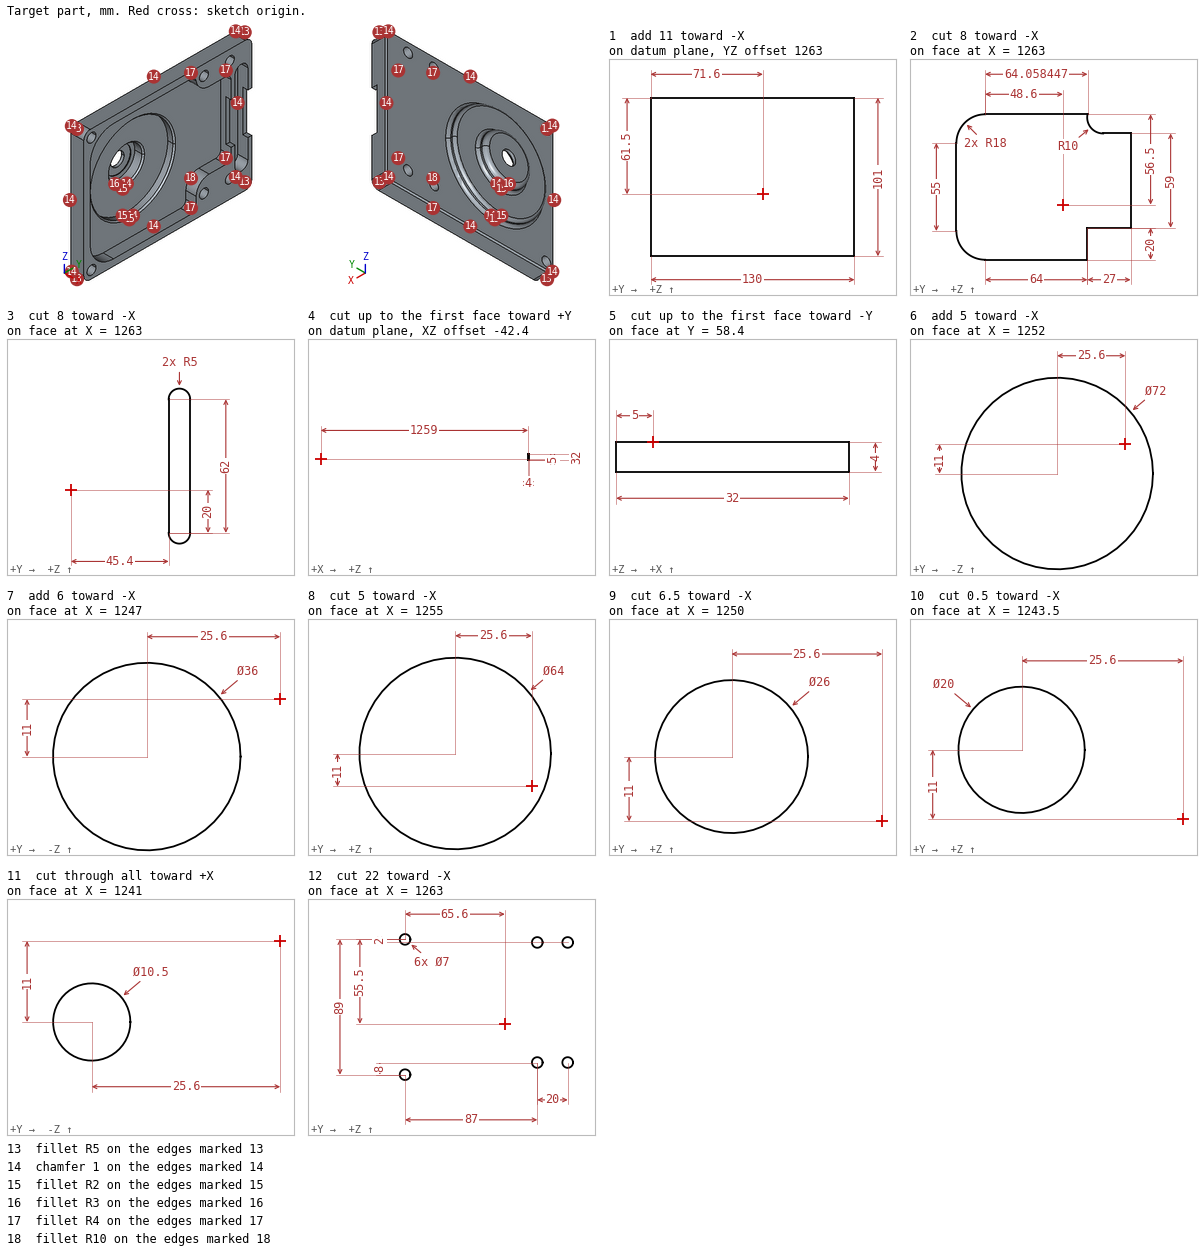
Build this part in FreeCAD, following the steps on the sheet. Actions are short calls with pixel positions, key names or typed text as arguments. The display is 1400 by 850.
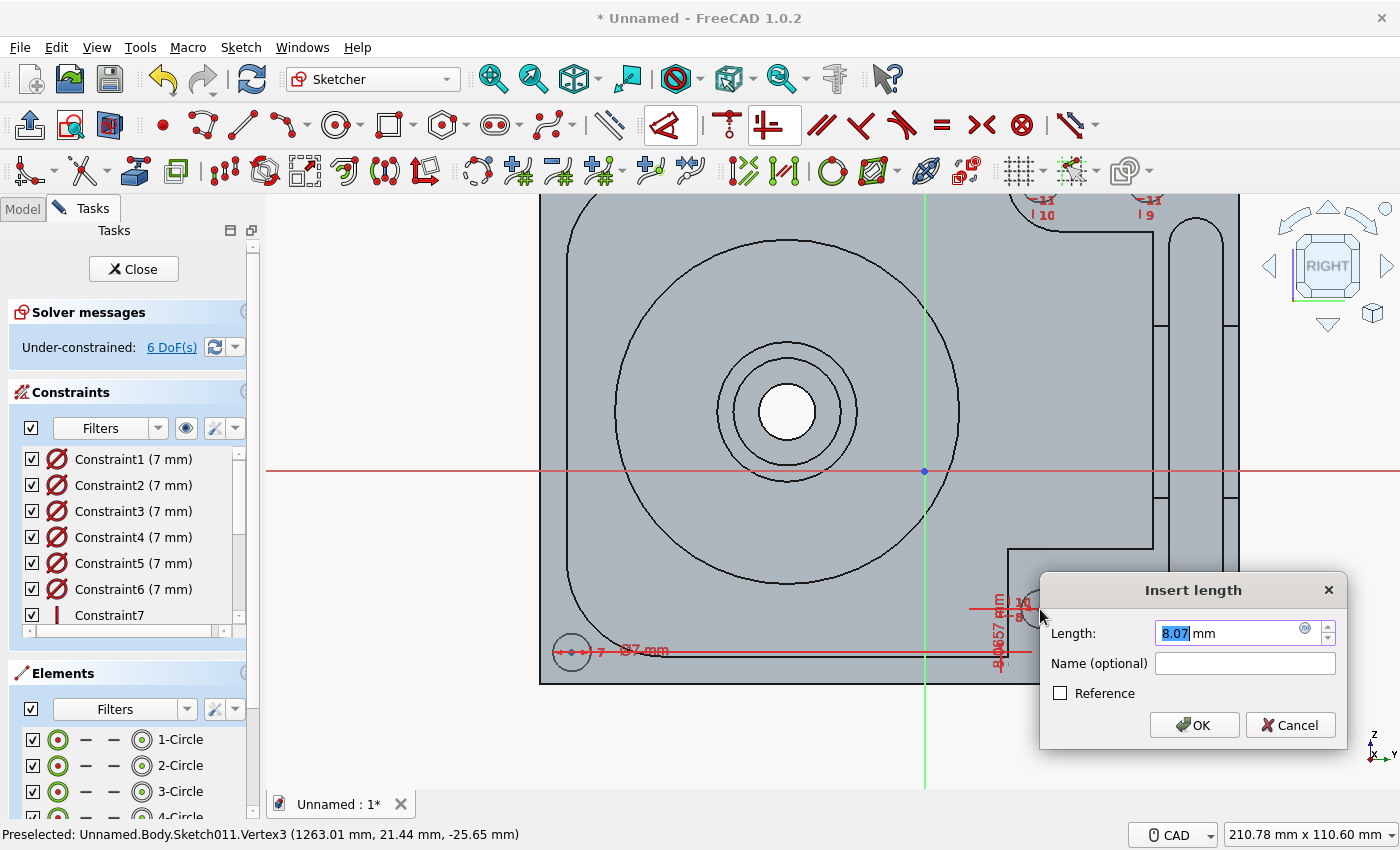
text(8)
key(Return)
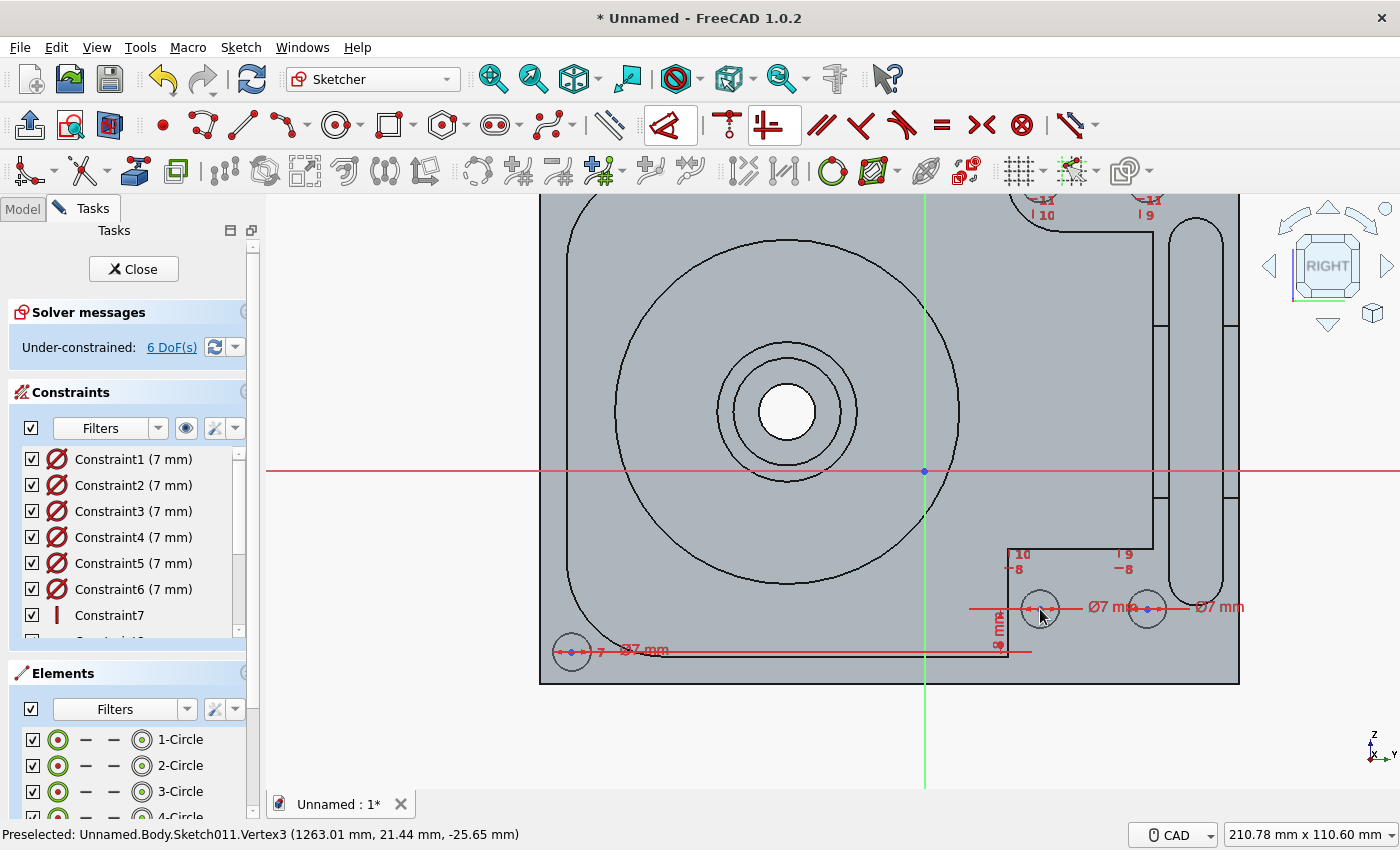
scroll(571, 653, down, 2)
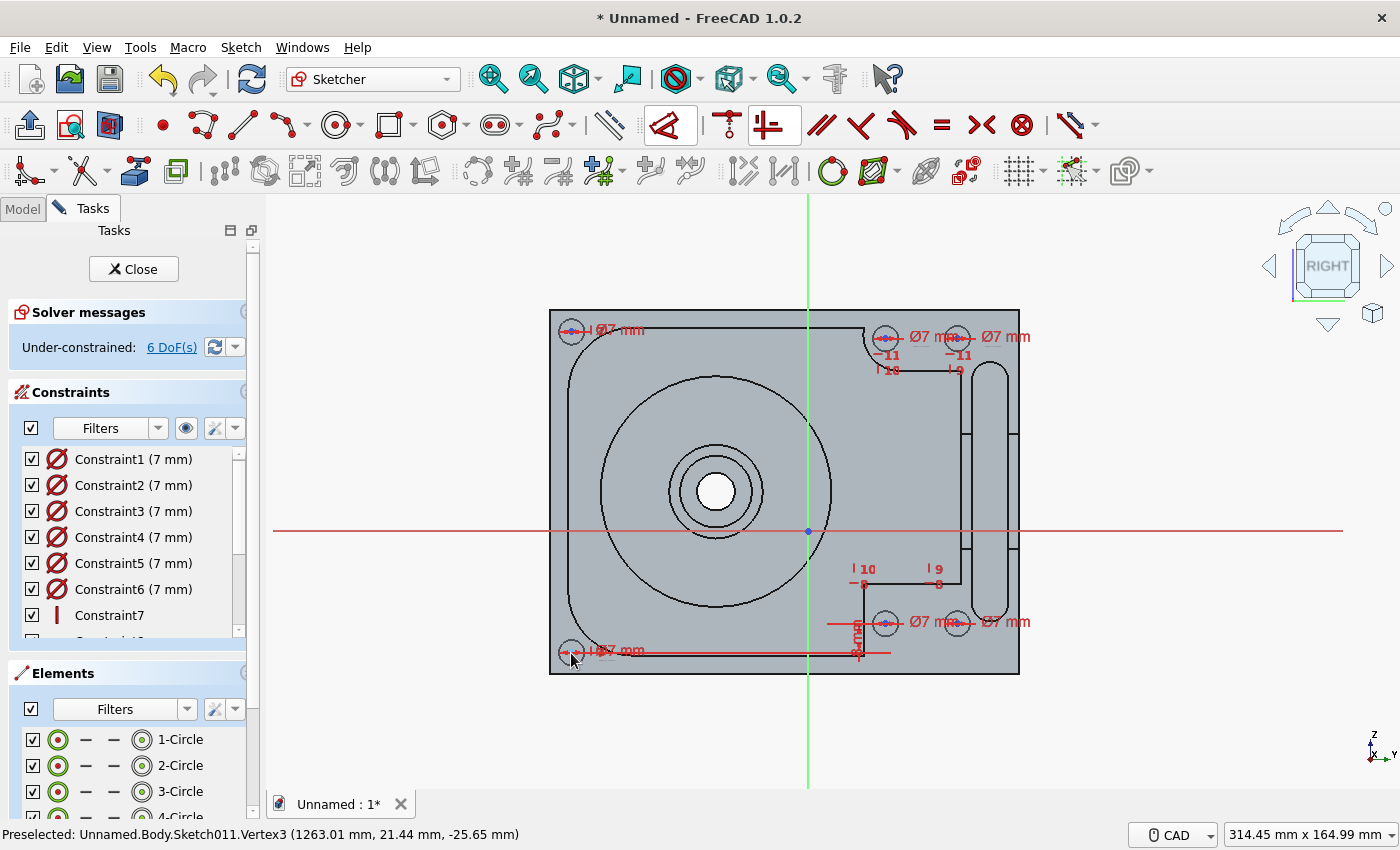
scroll(572, 332, up, 9)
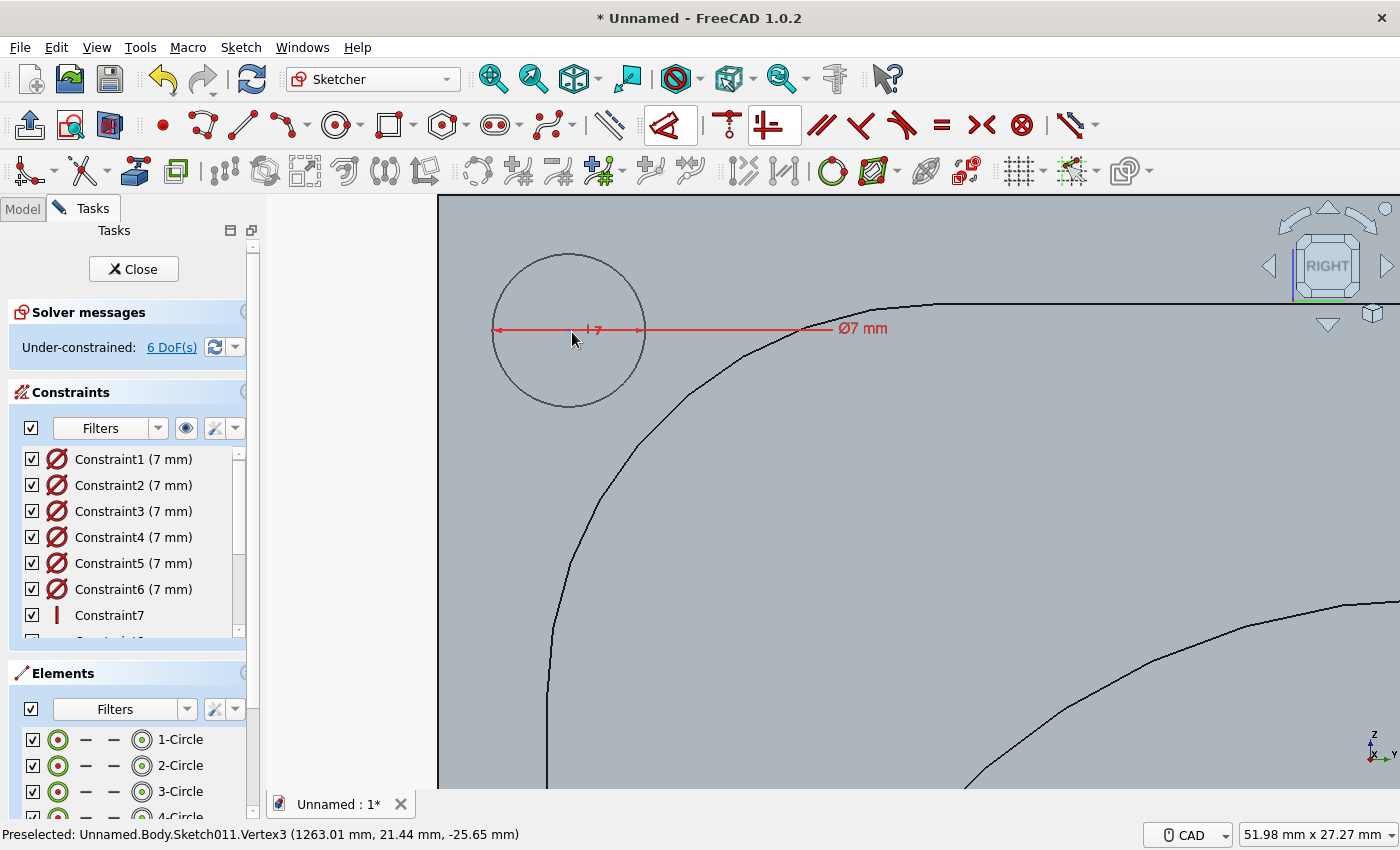
click(569, 330)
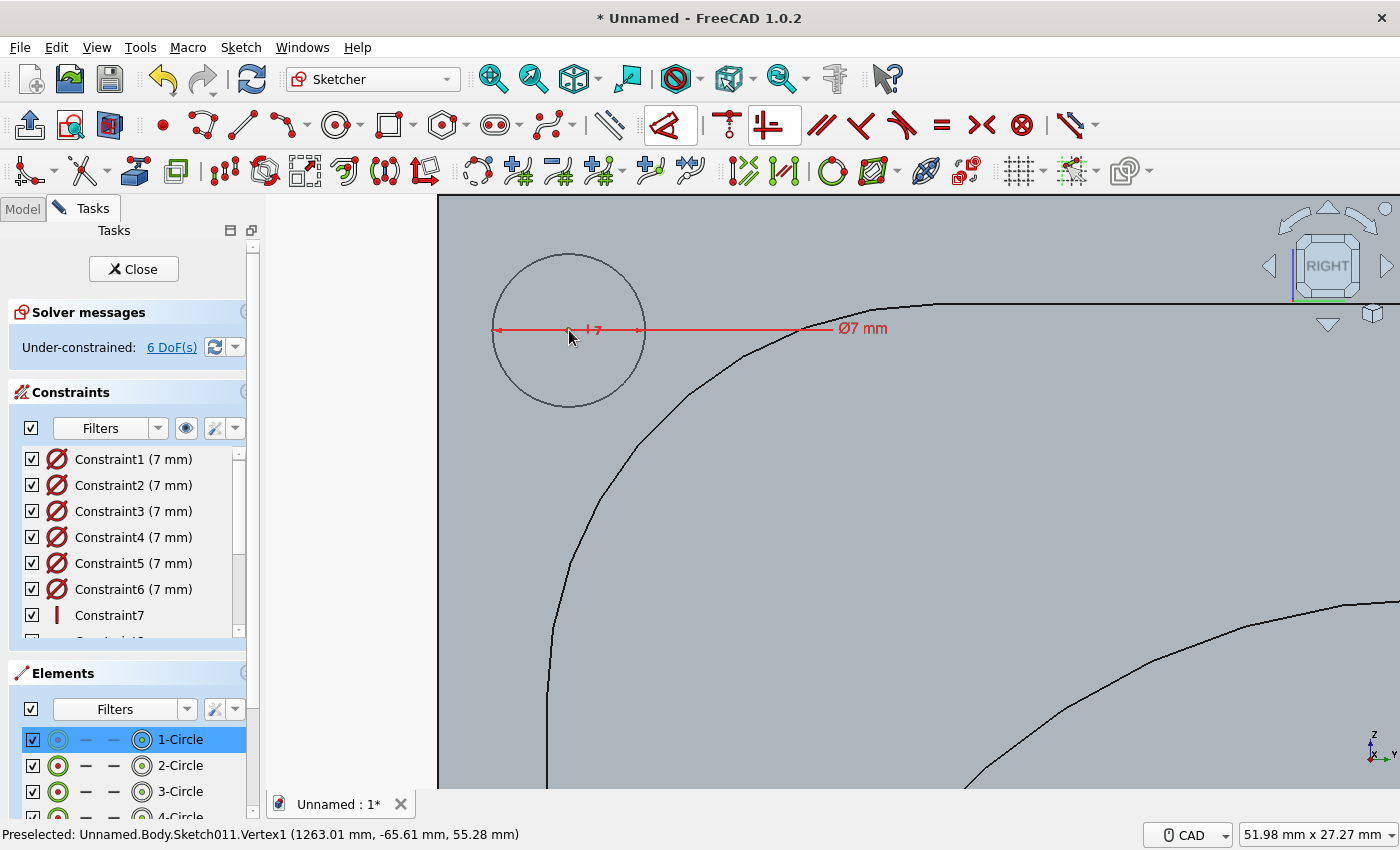
scroll(572, 332, down, 9)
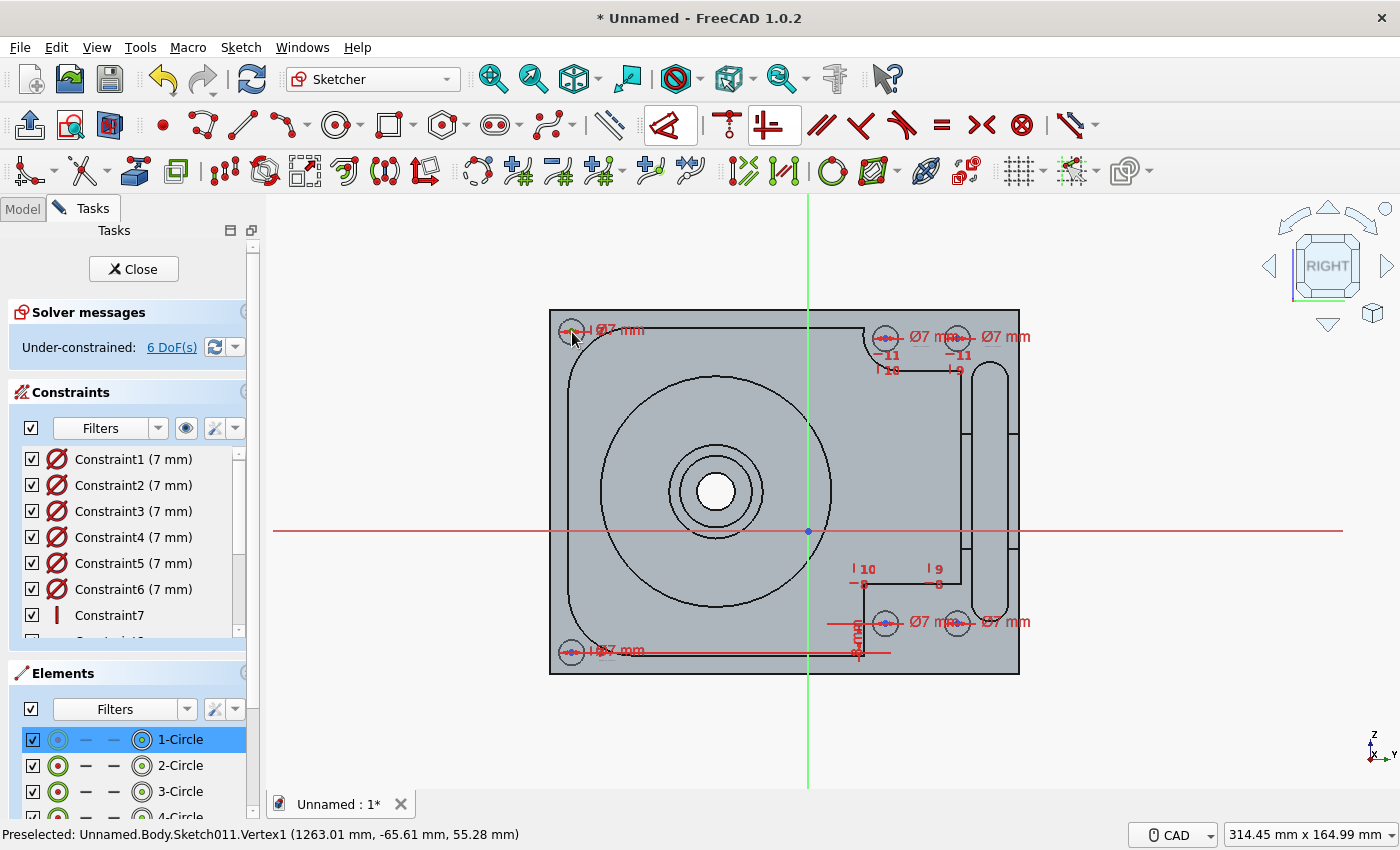
scroll(957, 339, up, 9)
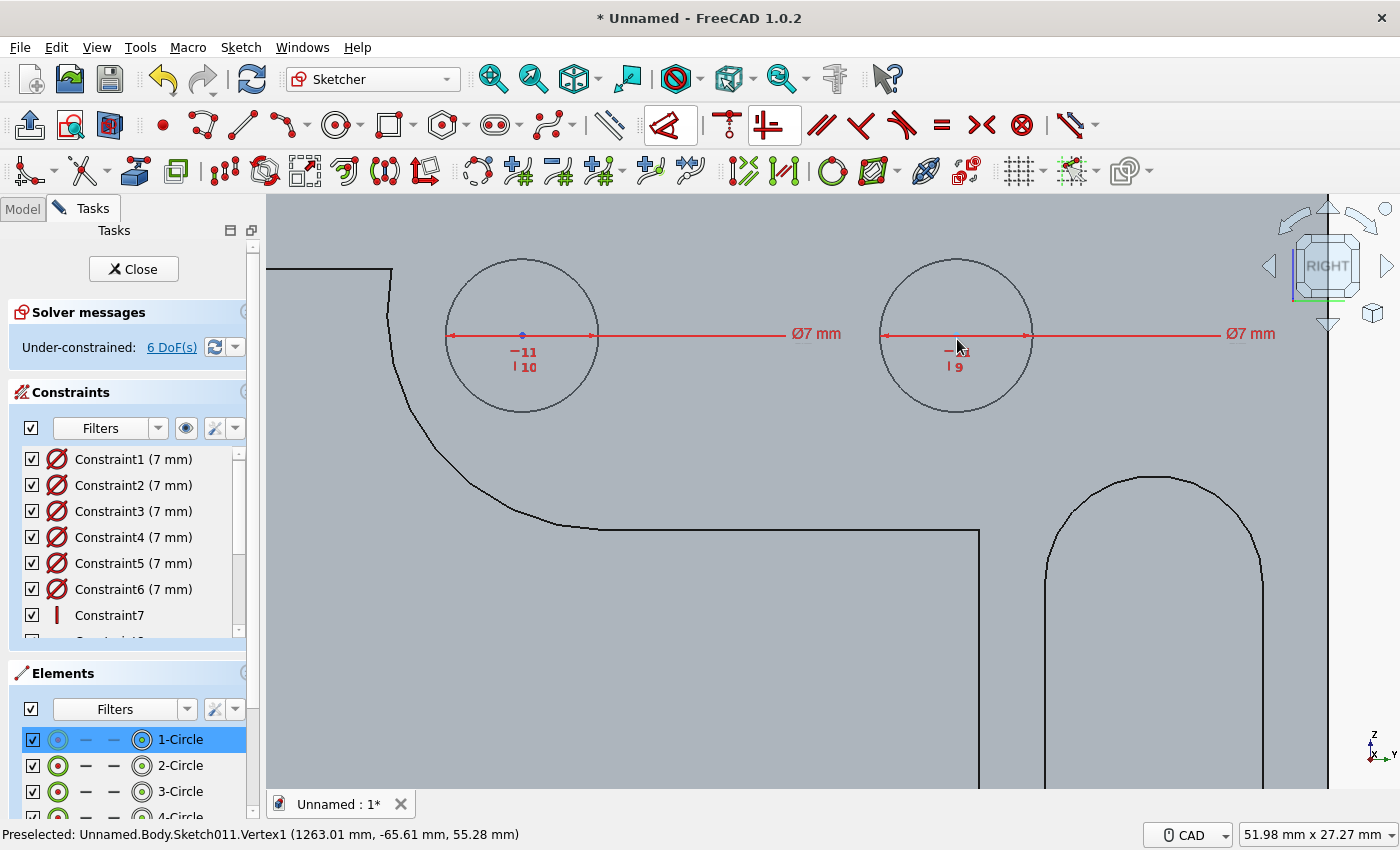
click(956, 336)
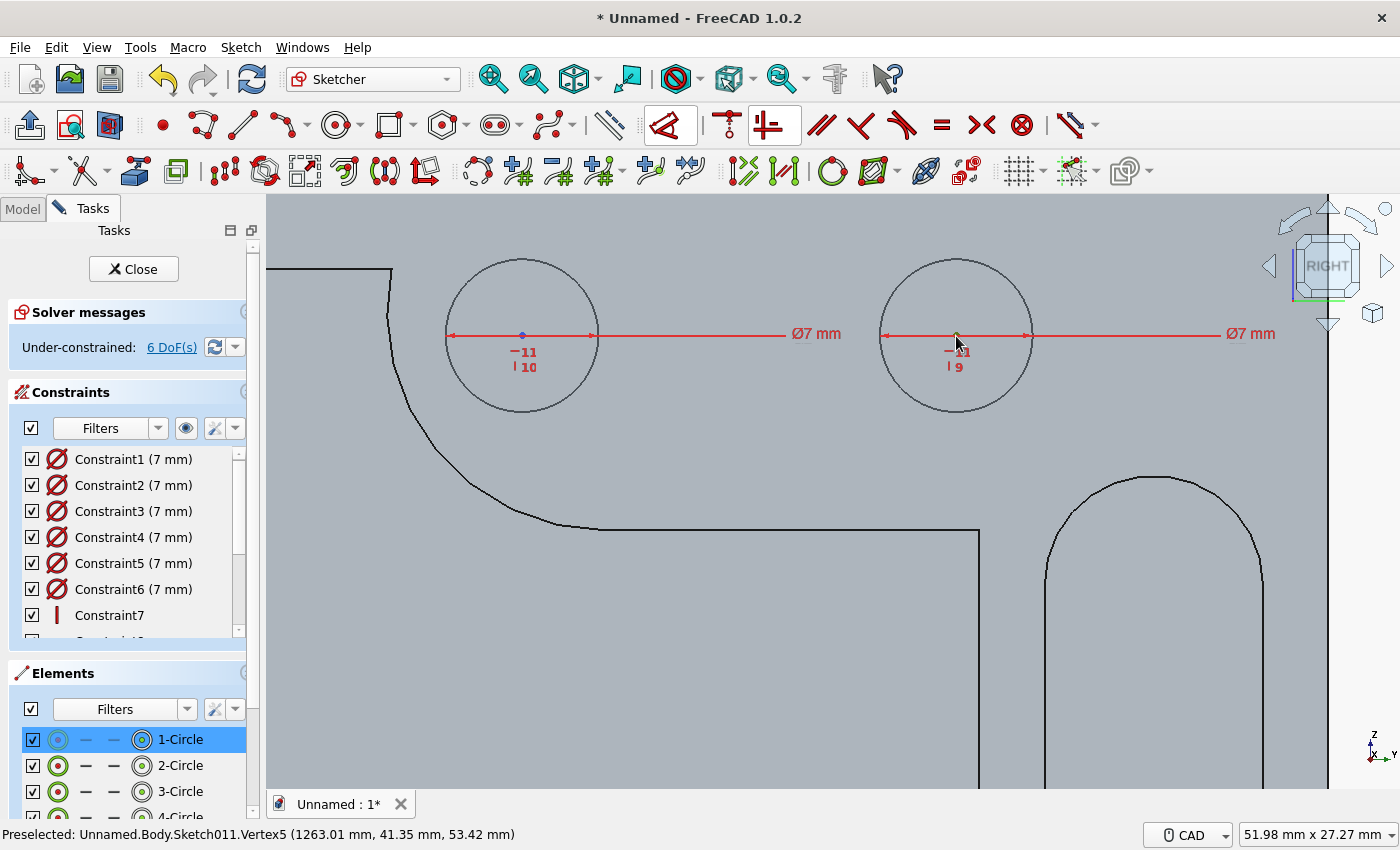
click(692, 126)